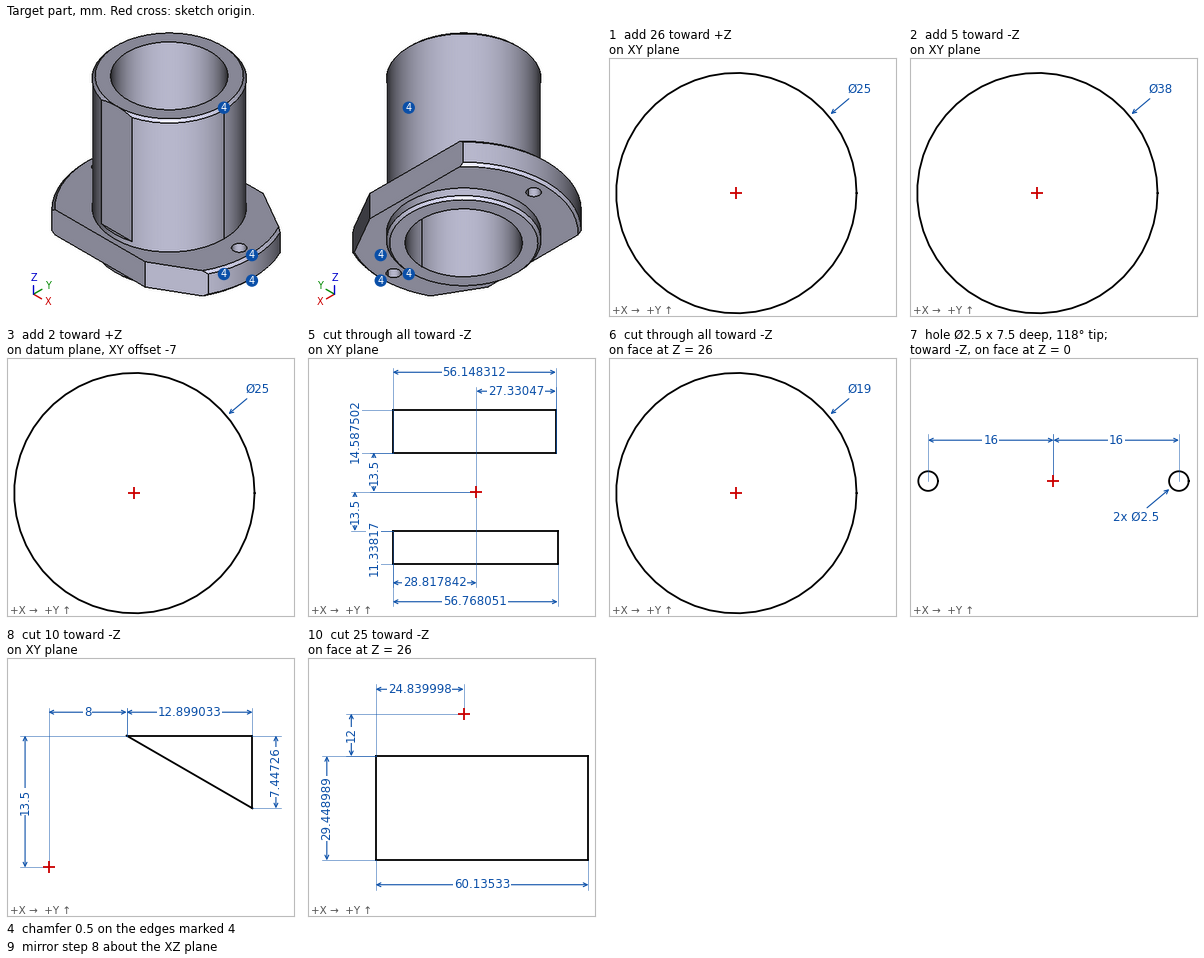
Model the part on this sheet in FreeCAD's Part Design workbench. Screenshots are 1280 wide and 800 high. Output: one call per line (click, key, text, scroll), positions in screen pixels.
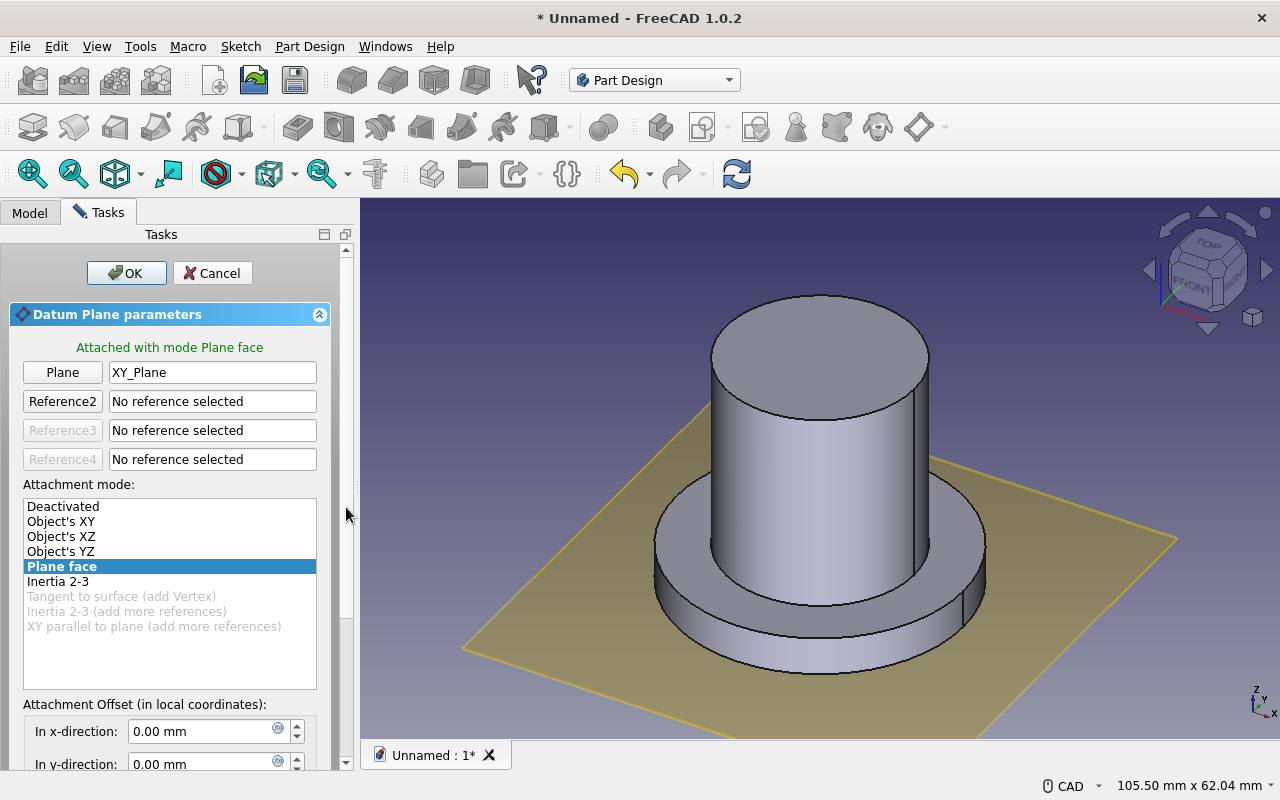
click(127, 273)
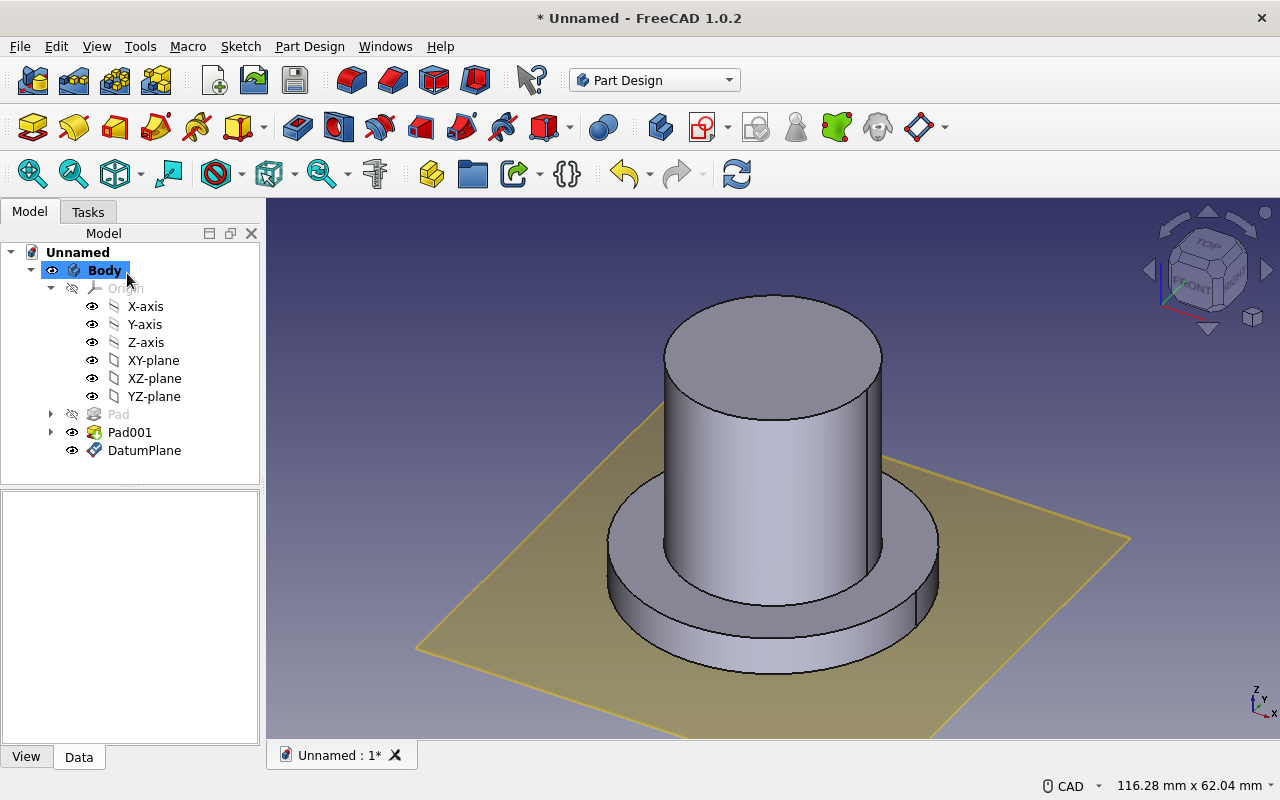
click(117, 450)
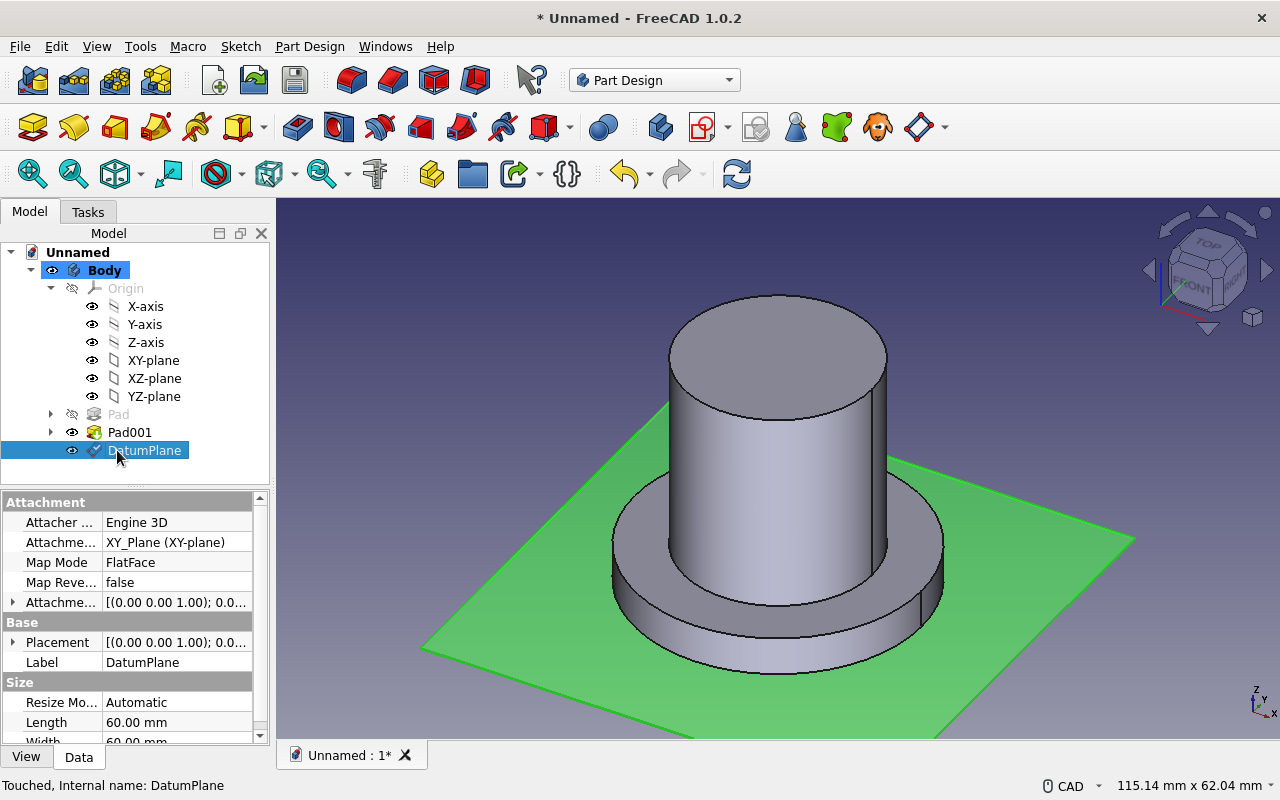
click(702, 128)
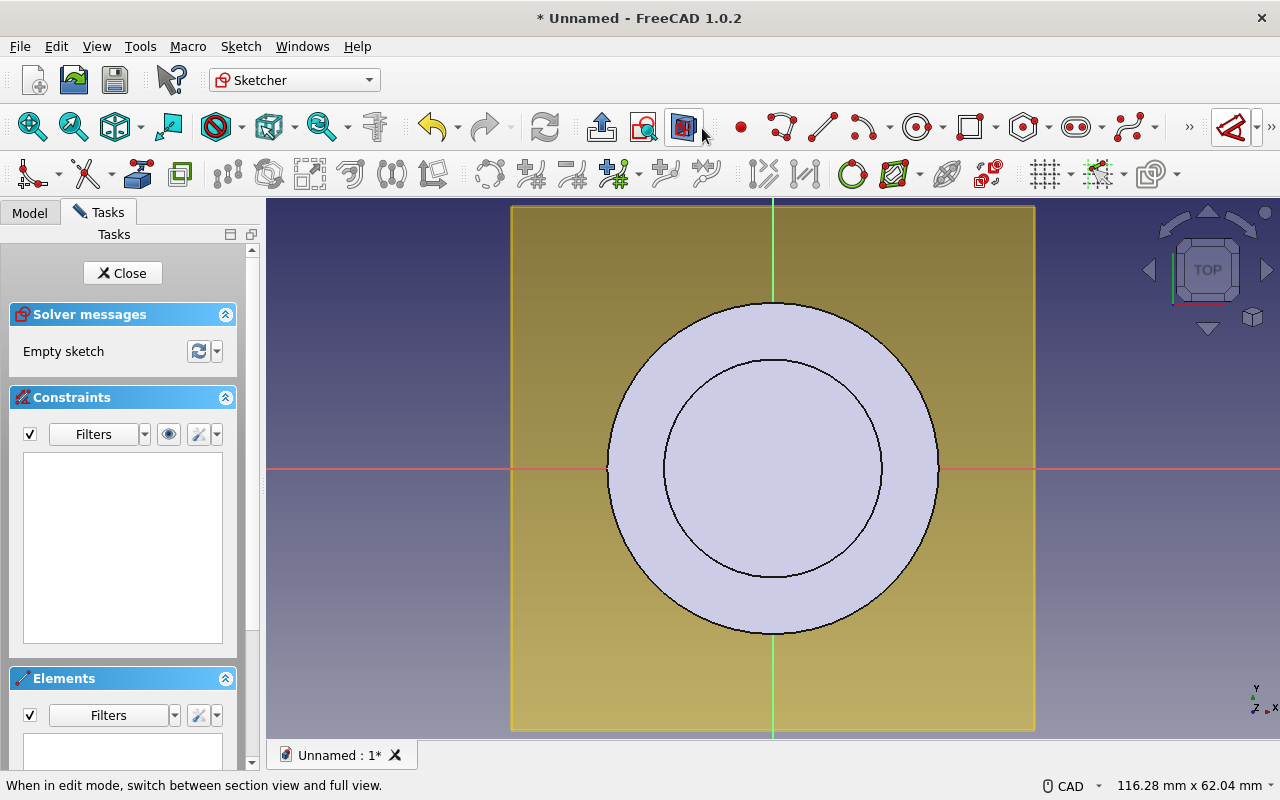
click(684, 128)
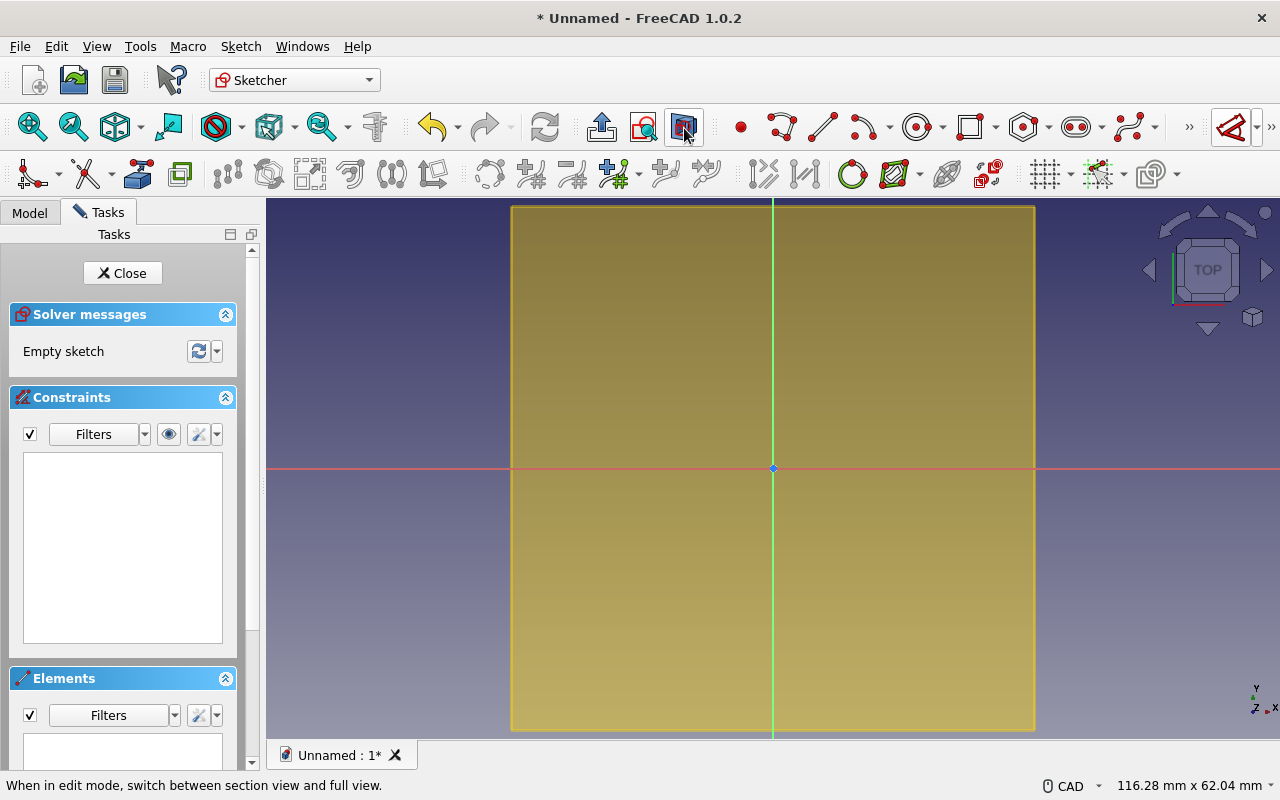
scroll(912, 469, up, 2)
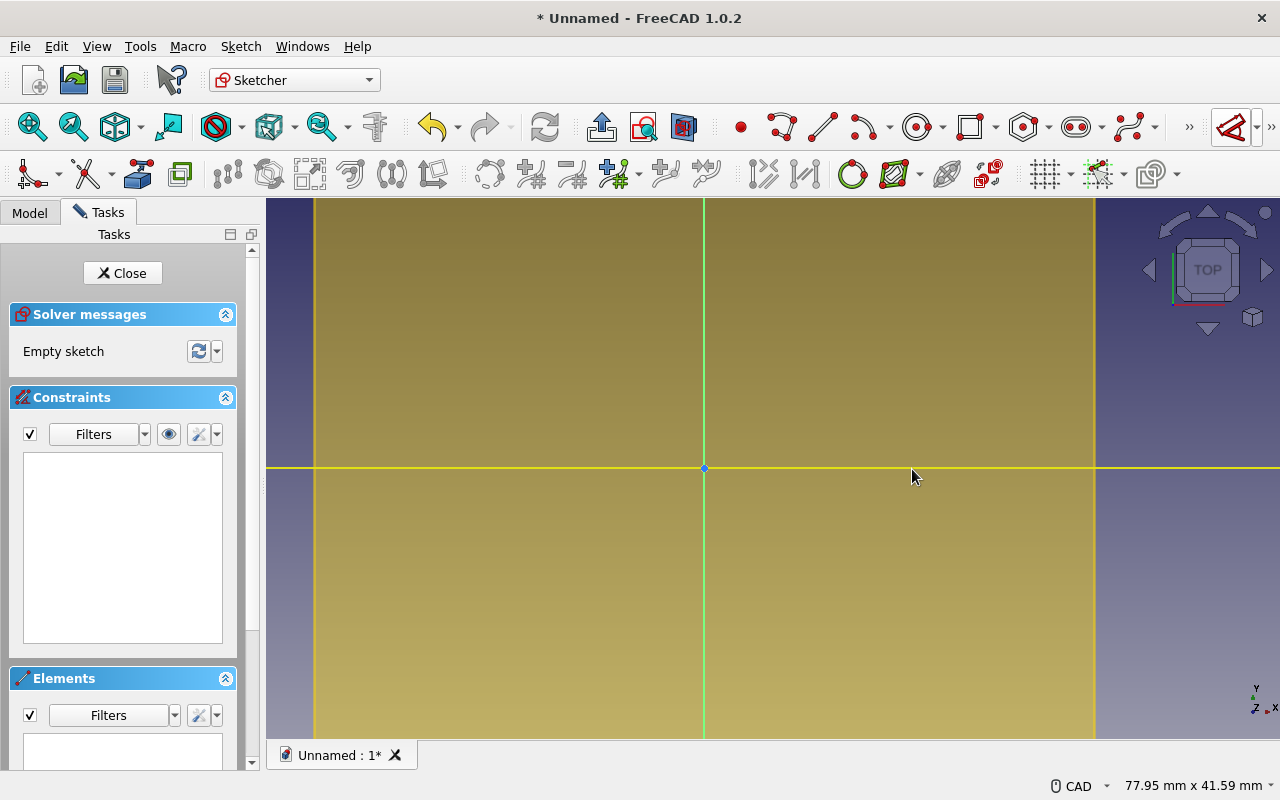
key(g)
key(c)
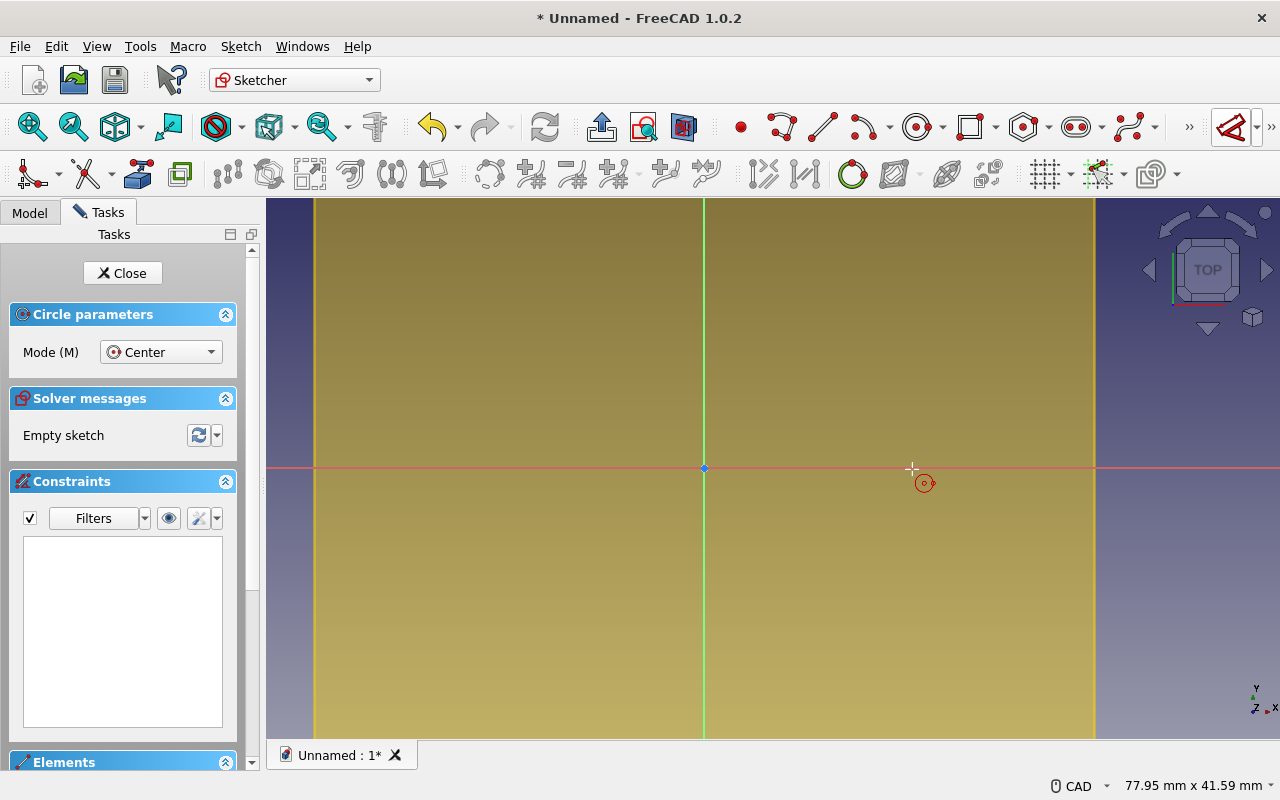
click(704, 468)
click(819, 353)
key(Escape)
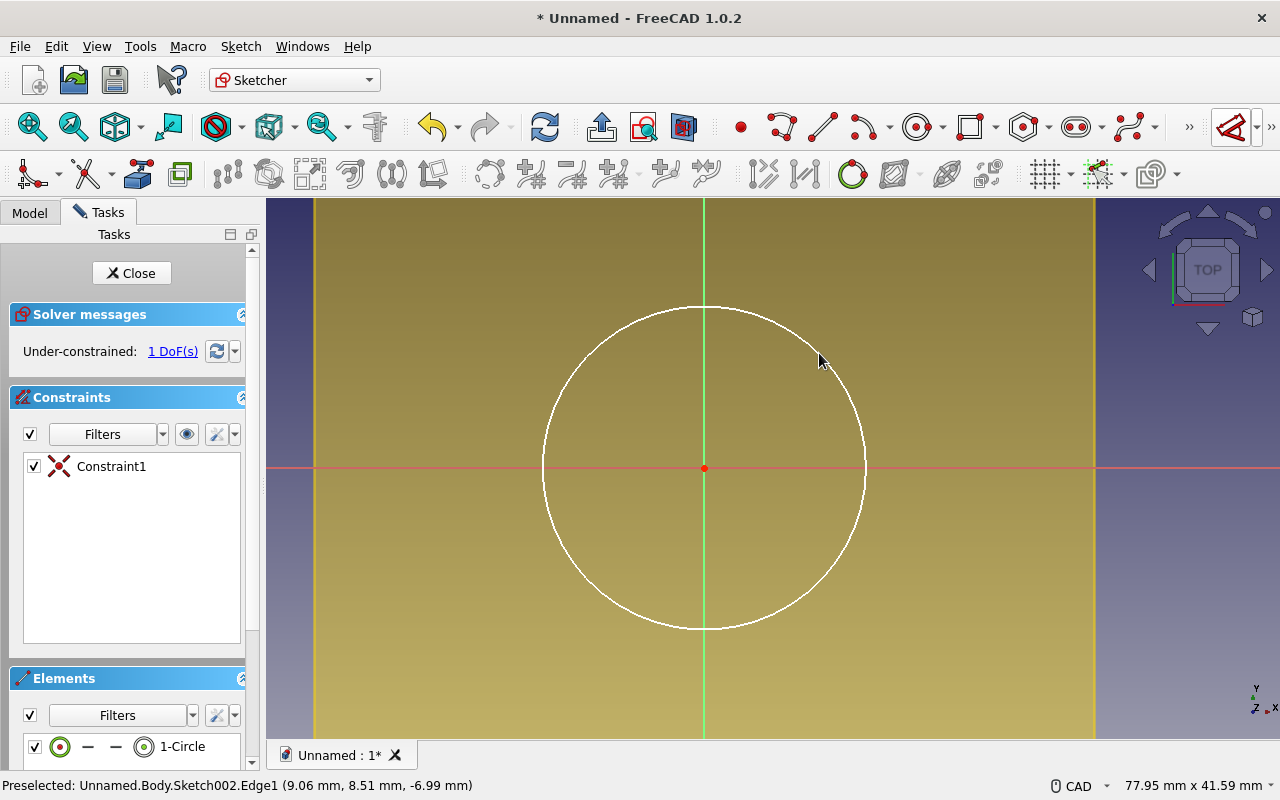
click(818, 353)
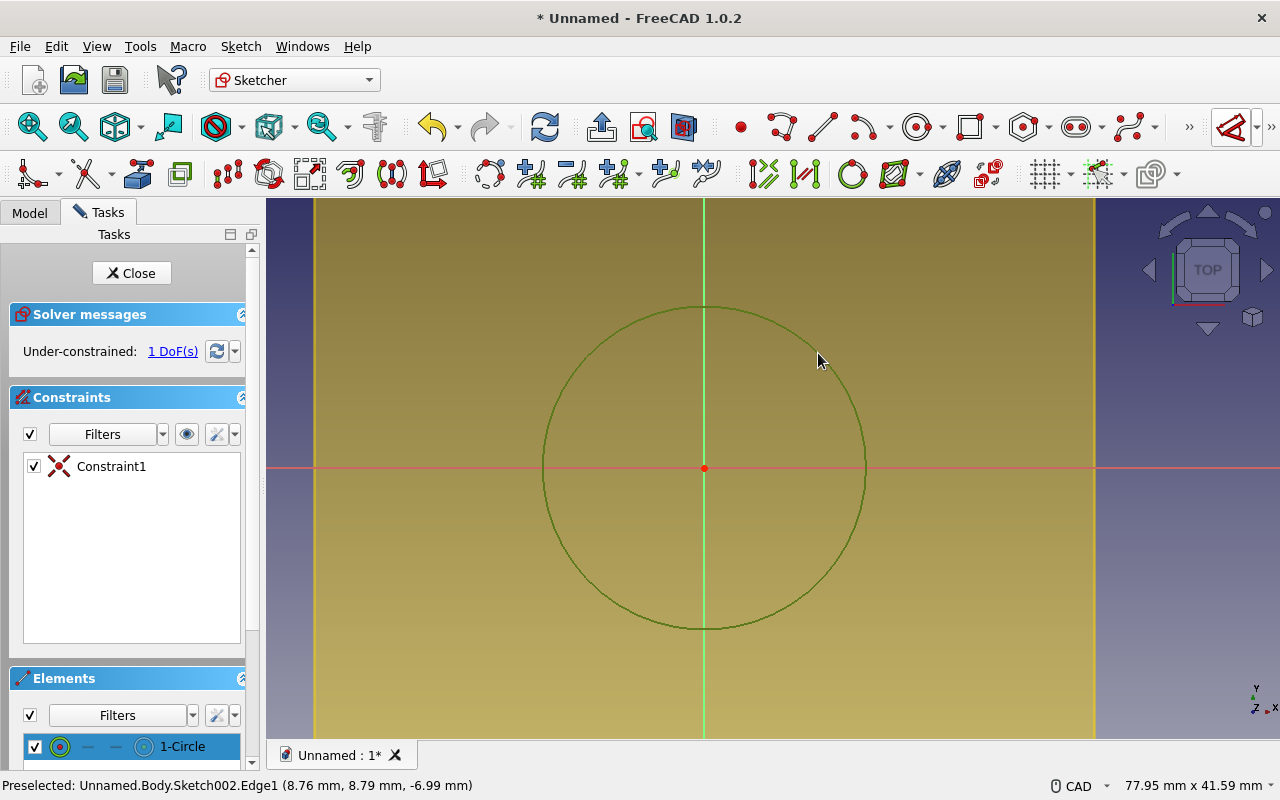
key(k)
key(o)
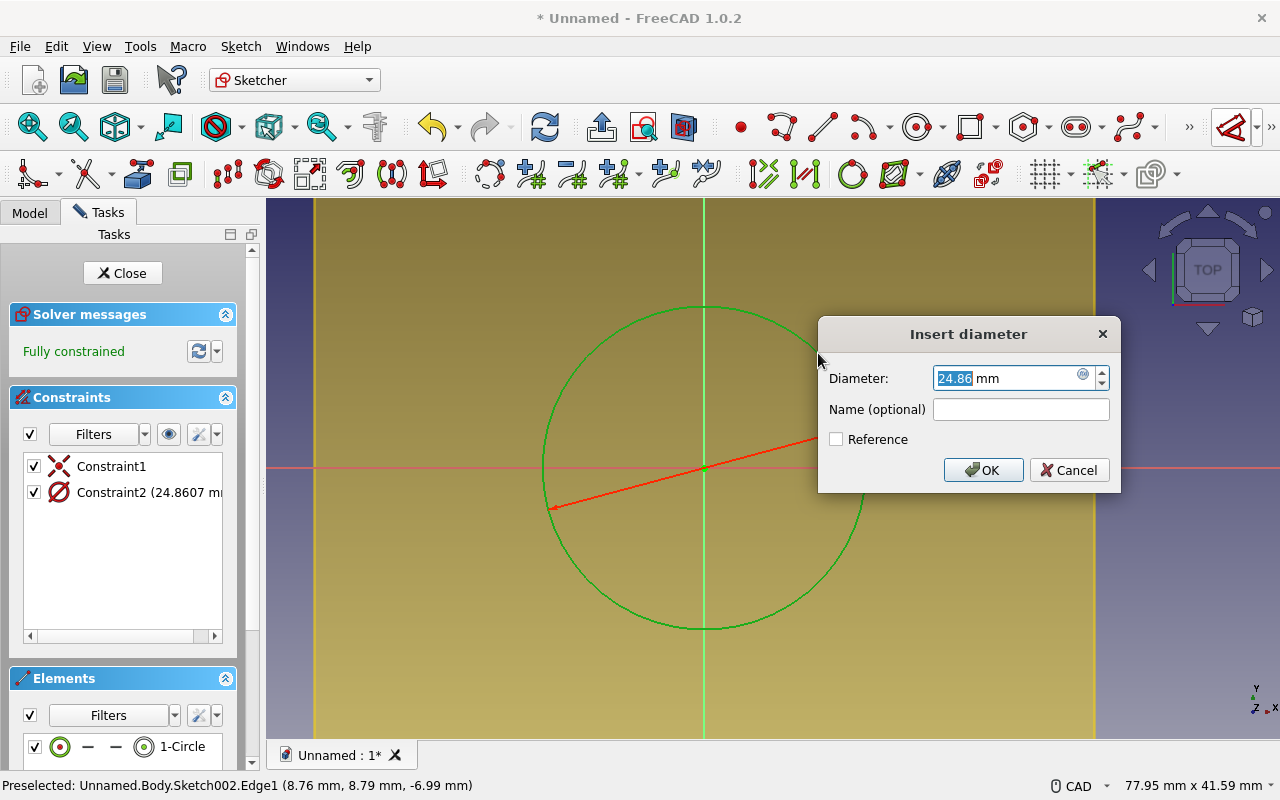
text(25)
key(Return)